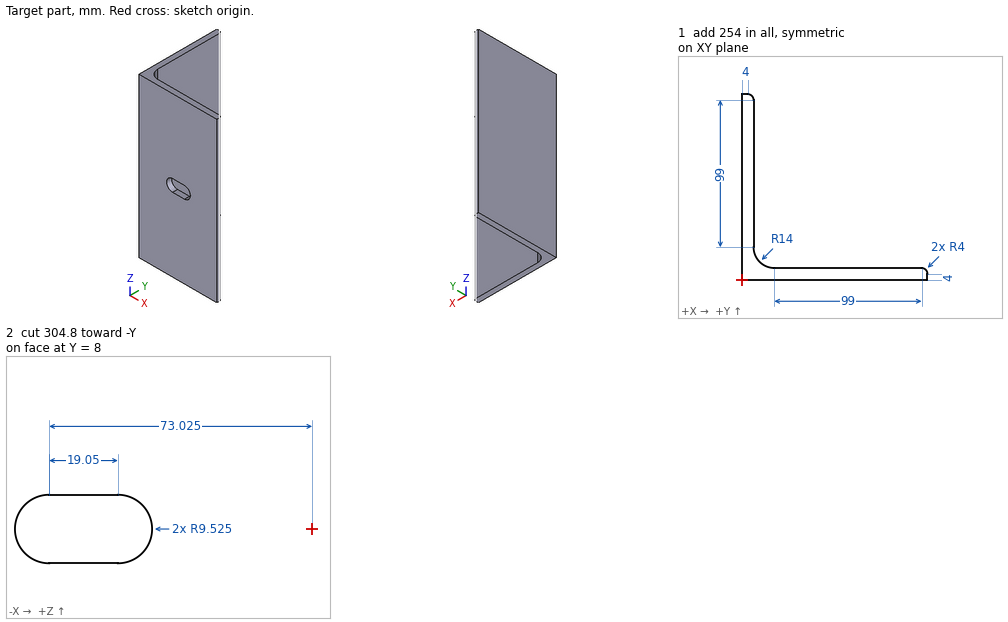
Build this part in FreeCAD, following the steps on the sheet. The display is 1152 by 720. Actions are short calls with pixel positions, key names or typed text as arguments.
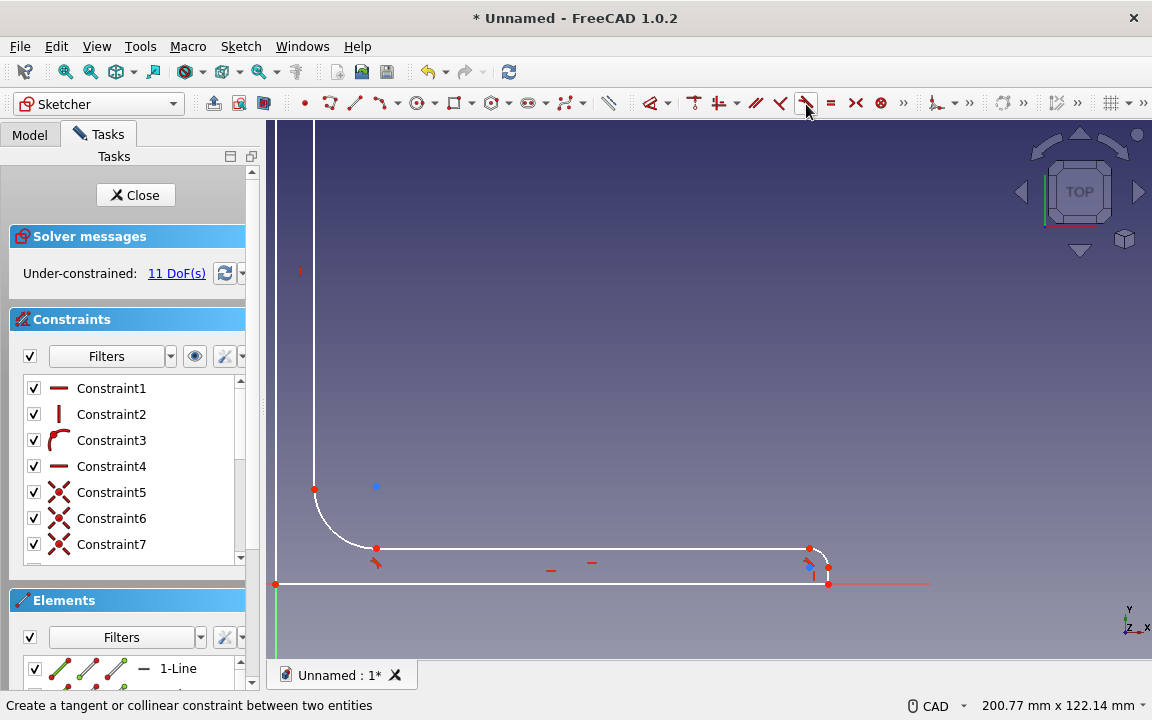
click(314, 358)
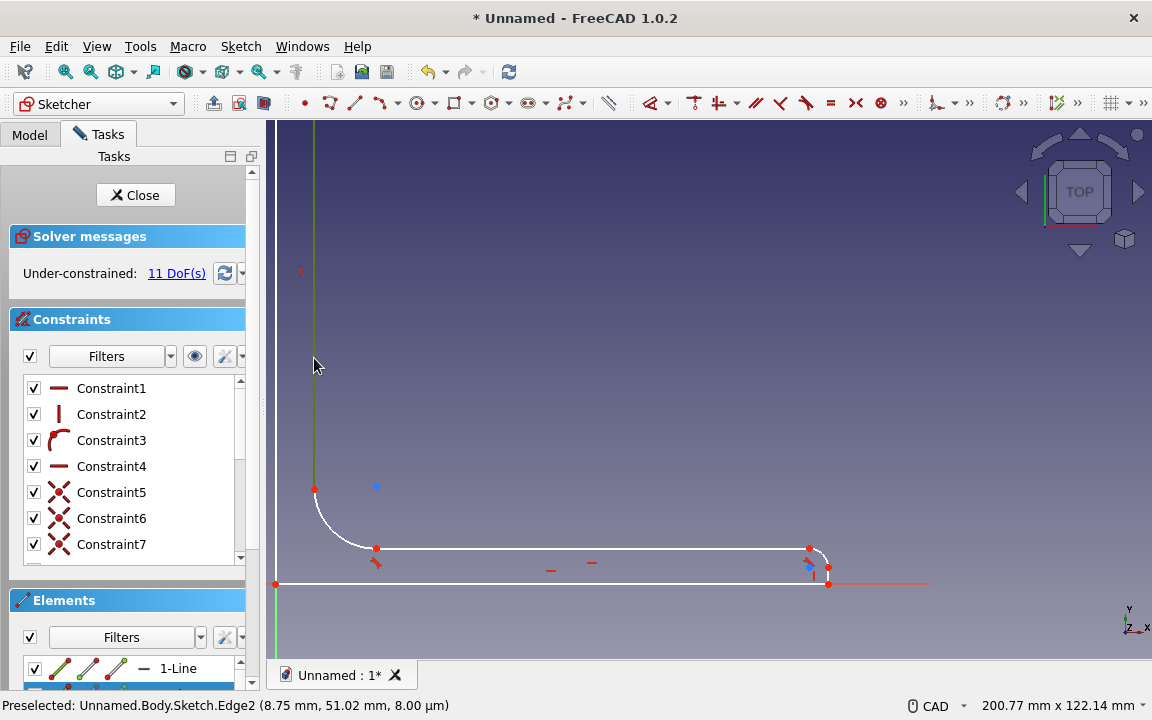
click(322, 516)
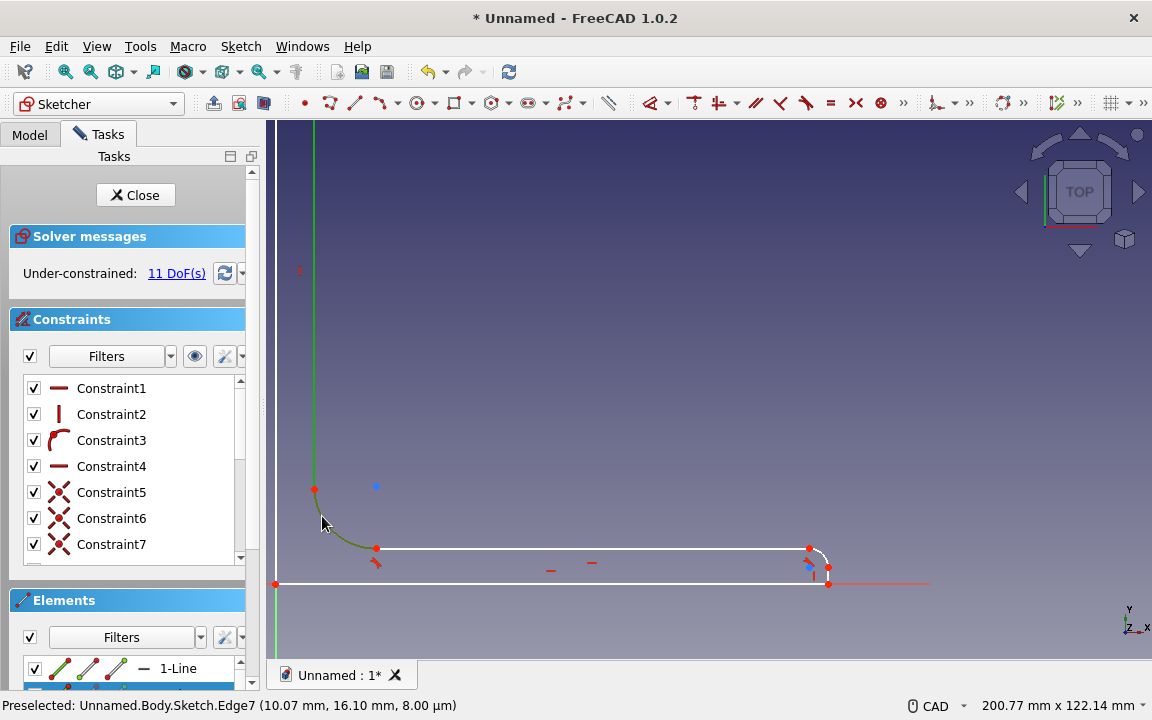
key(t)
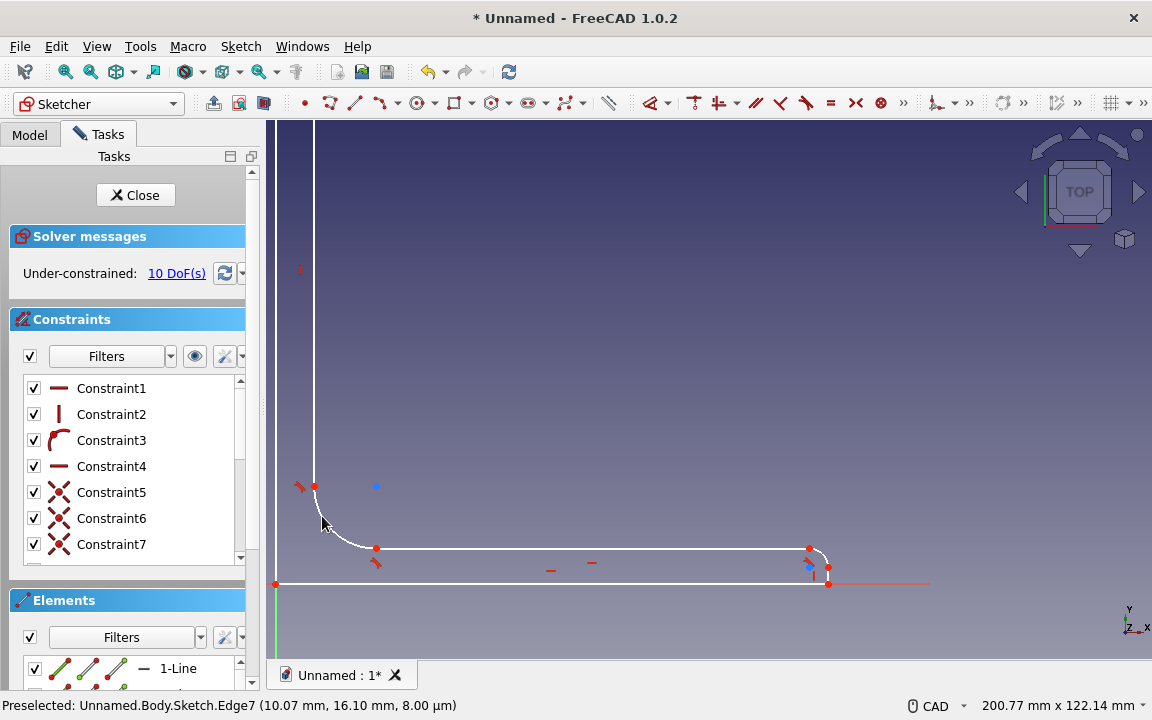
click(314, 356)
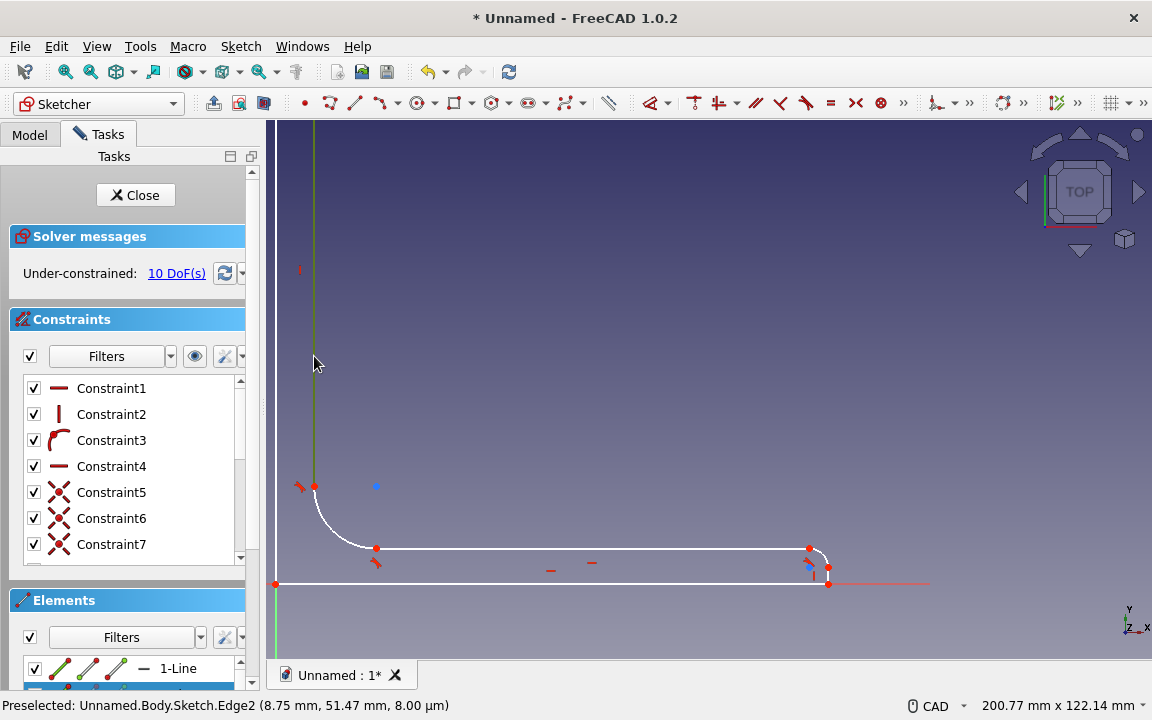
scroll(822, 555, down, 2)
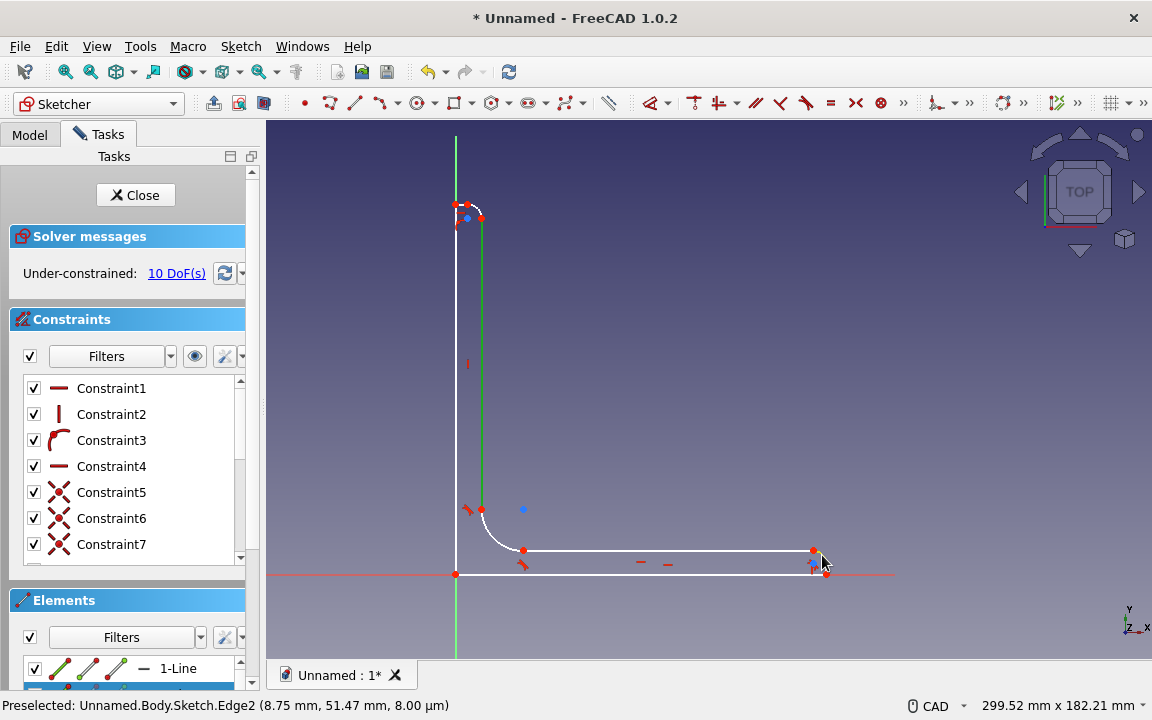
scroll(480, 212, up, 4)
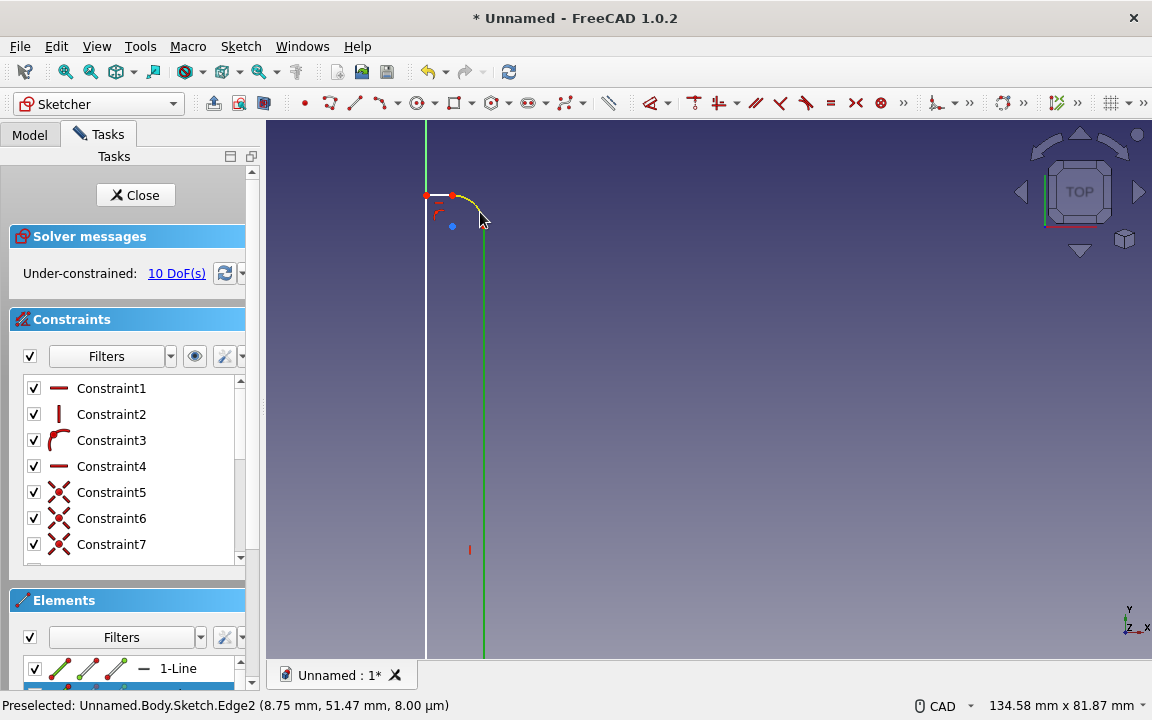
click(480, 212)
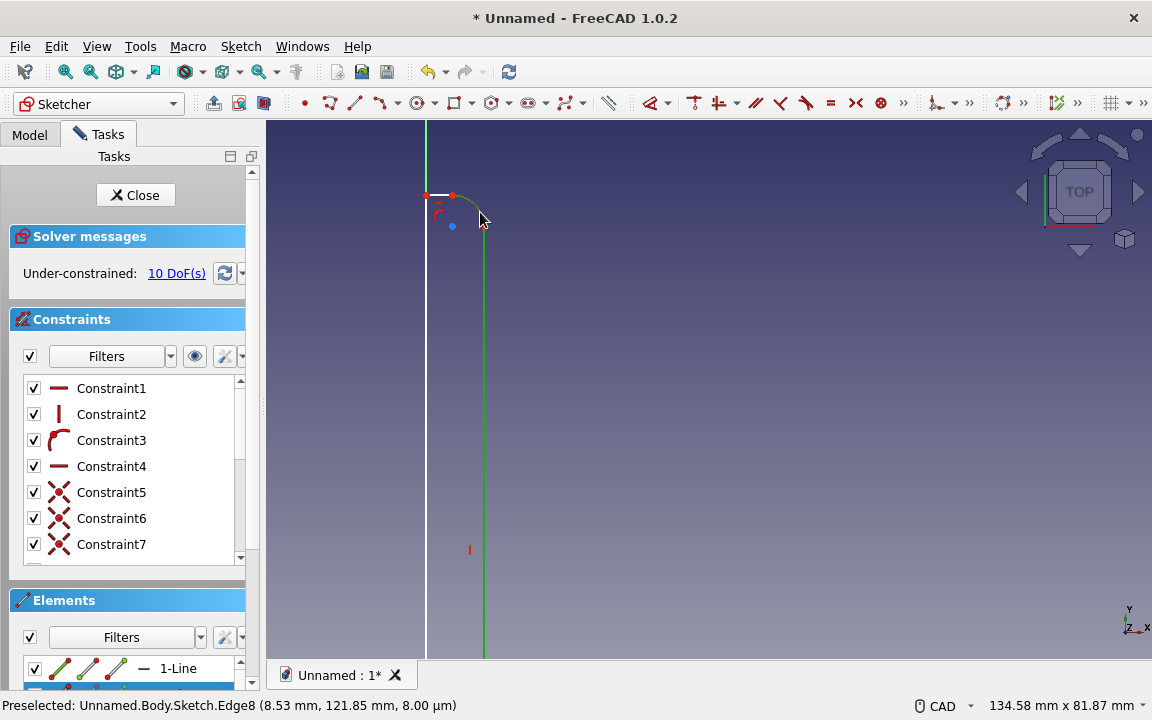
key(t)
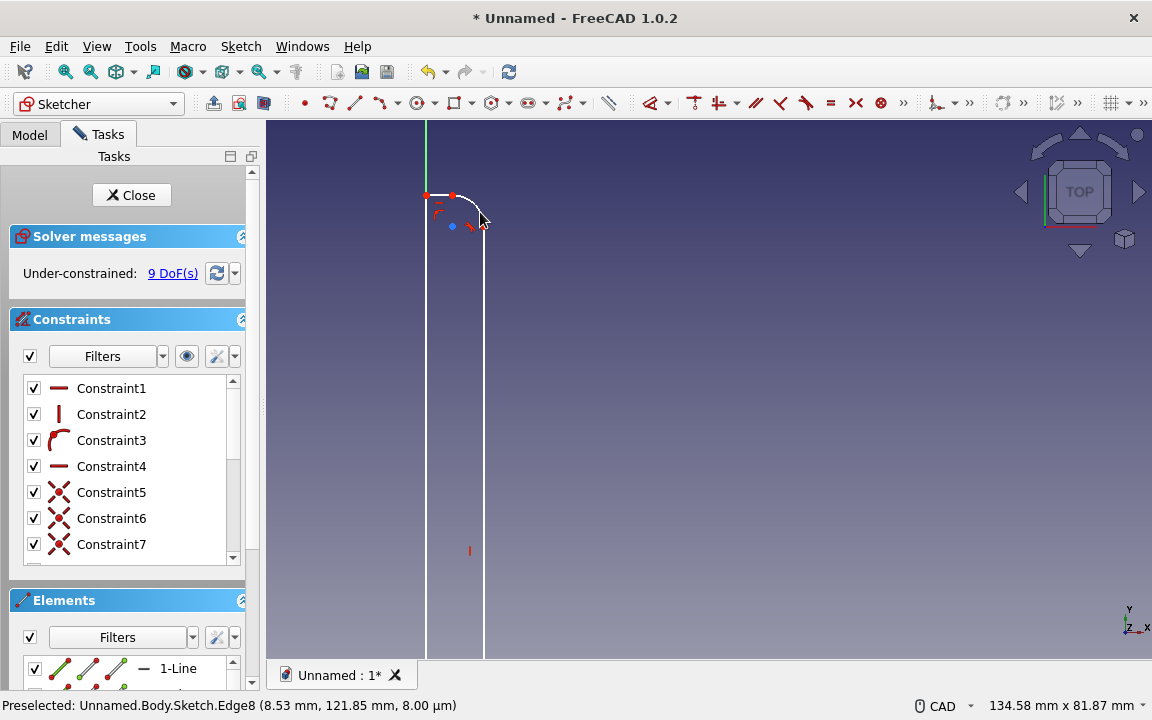
scroll(442, 195, up, 2)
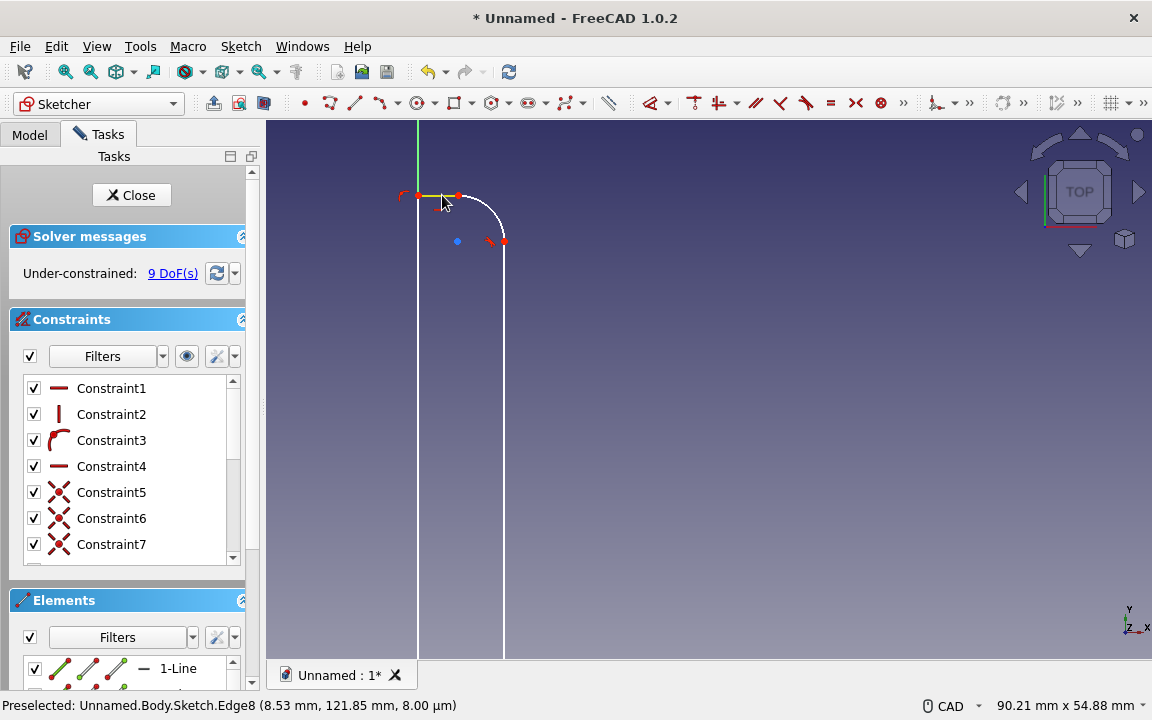
click(442, 196)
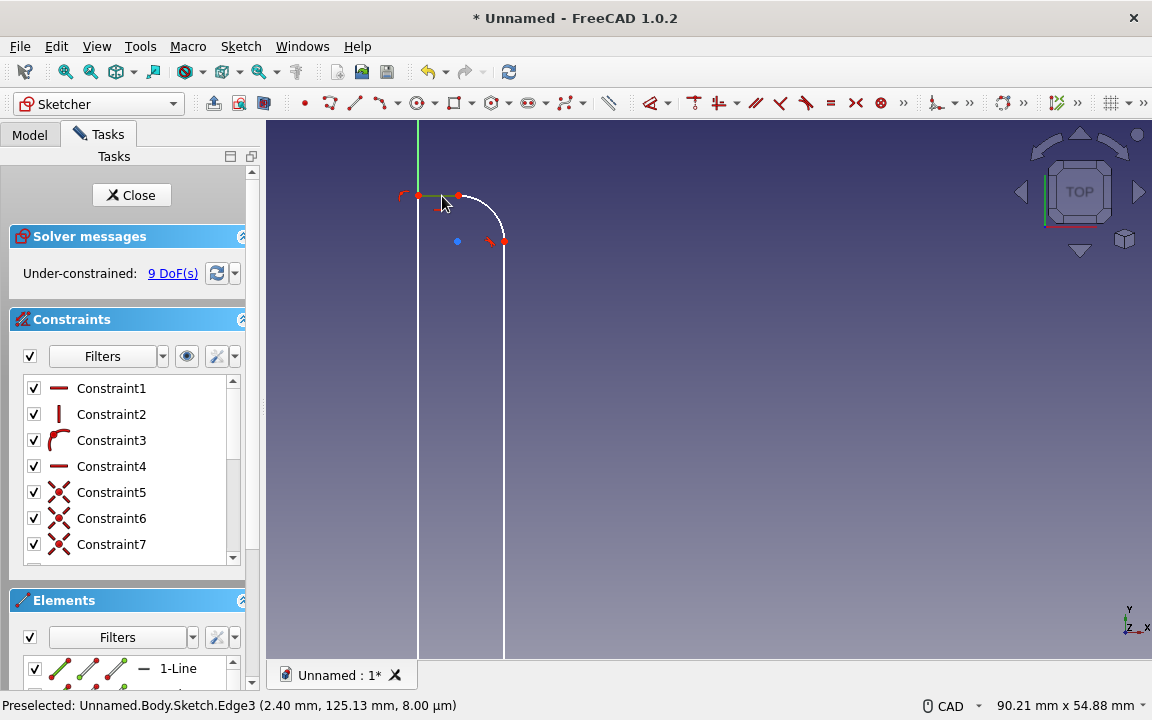
click(499, 221)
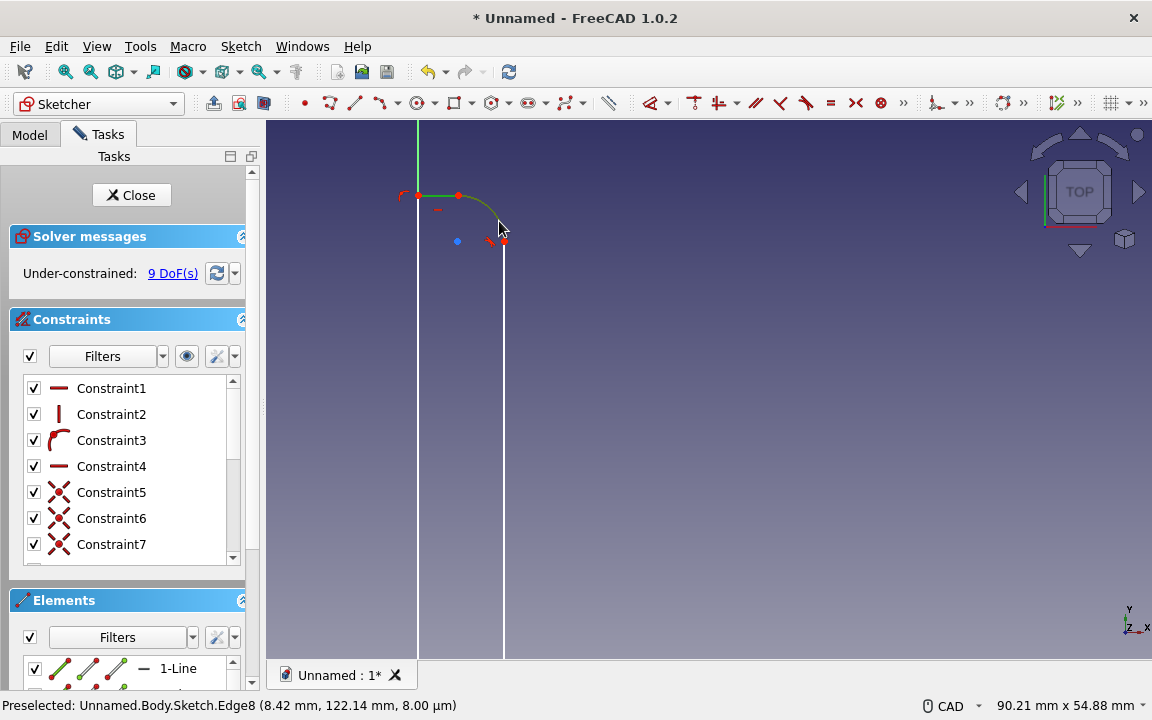
click(806, 104)